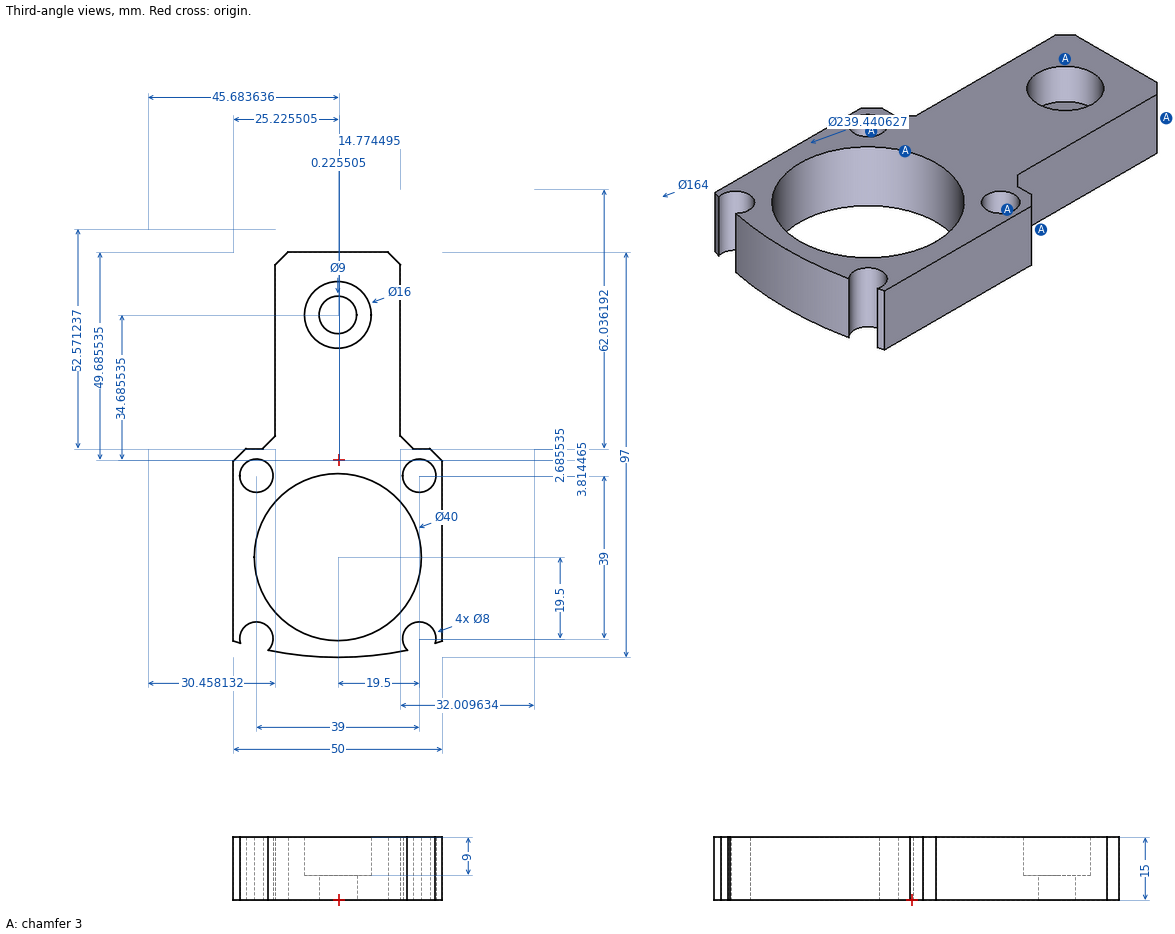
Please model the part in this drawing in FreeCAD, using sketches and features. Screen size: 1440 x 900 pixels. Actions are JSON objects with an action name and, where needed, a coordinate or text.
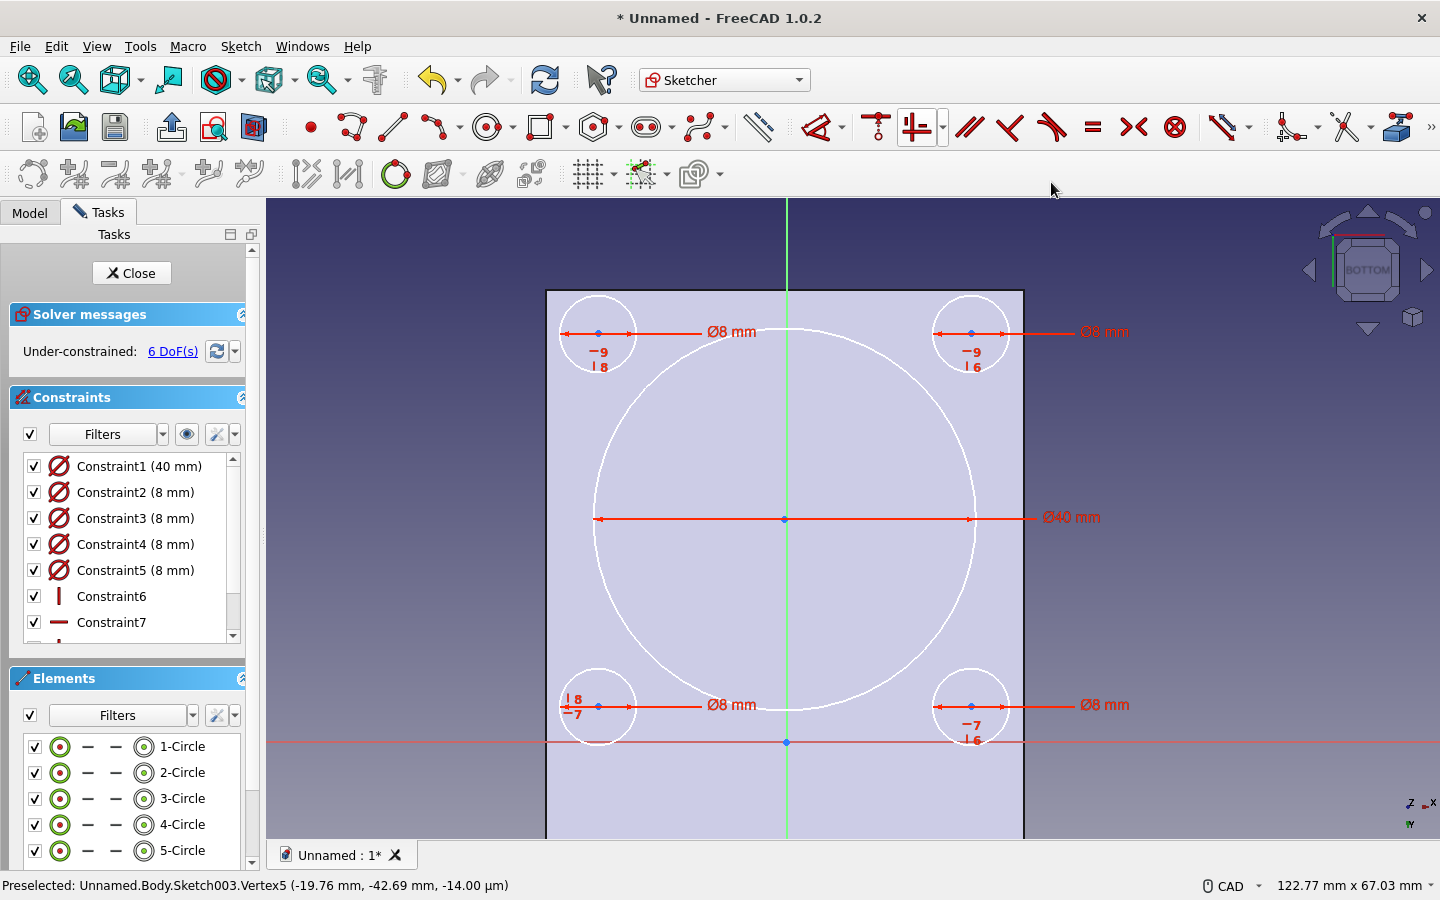
{"action": "left_click", "coordinate": [971, 334]}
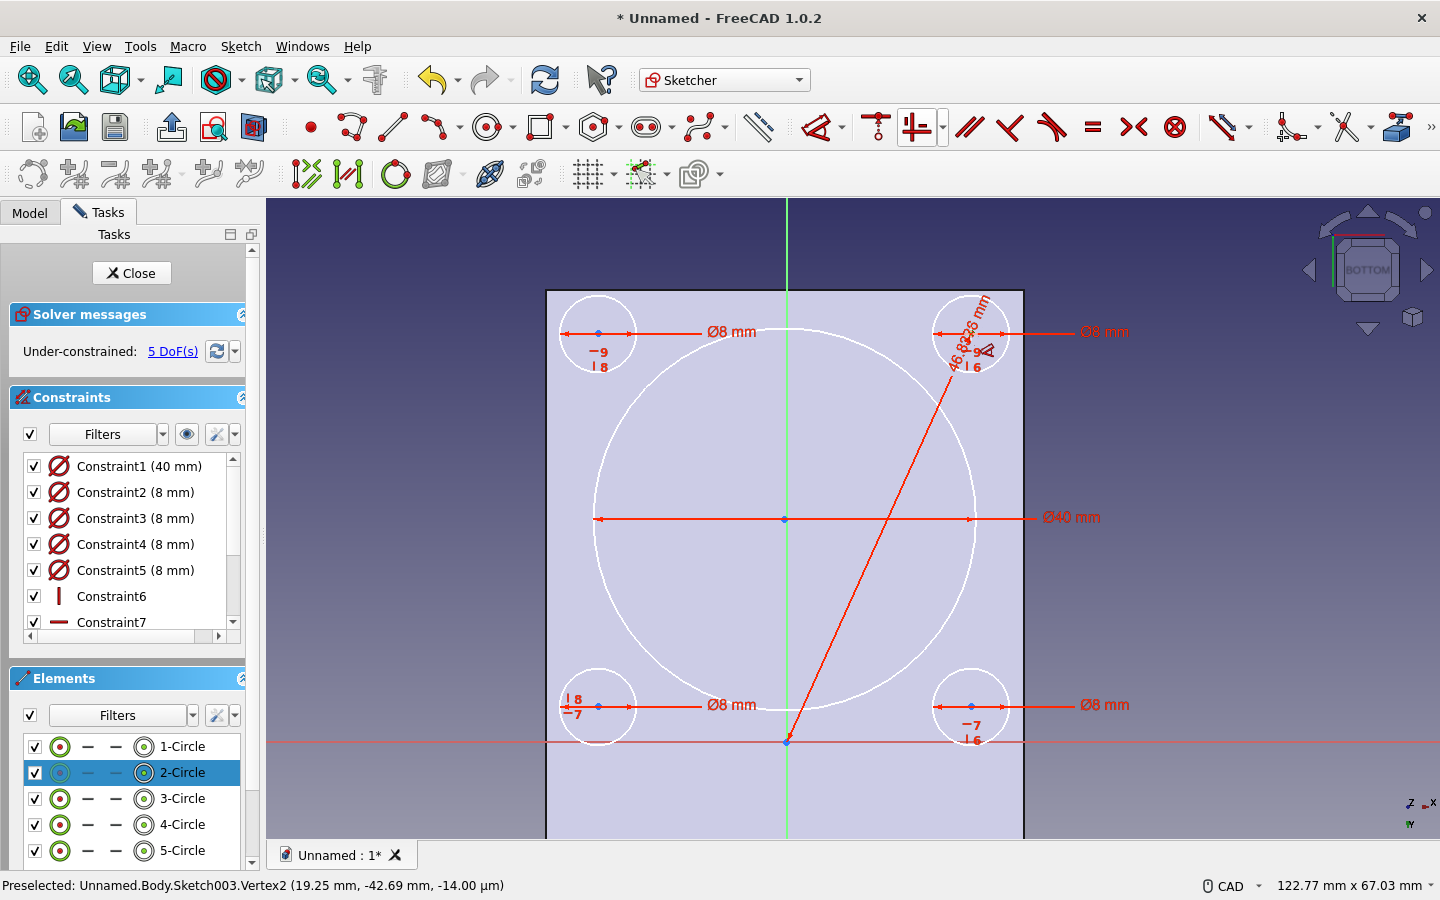
{"action": "left_click", "coordinate": [971, 707]}
{"action": "left_click", "coordinate": [1005, 521]}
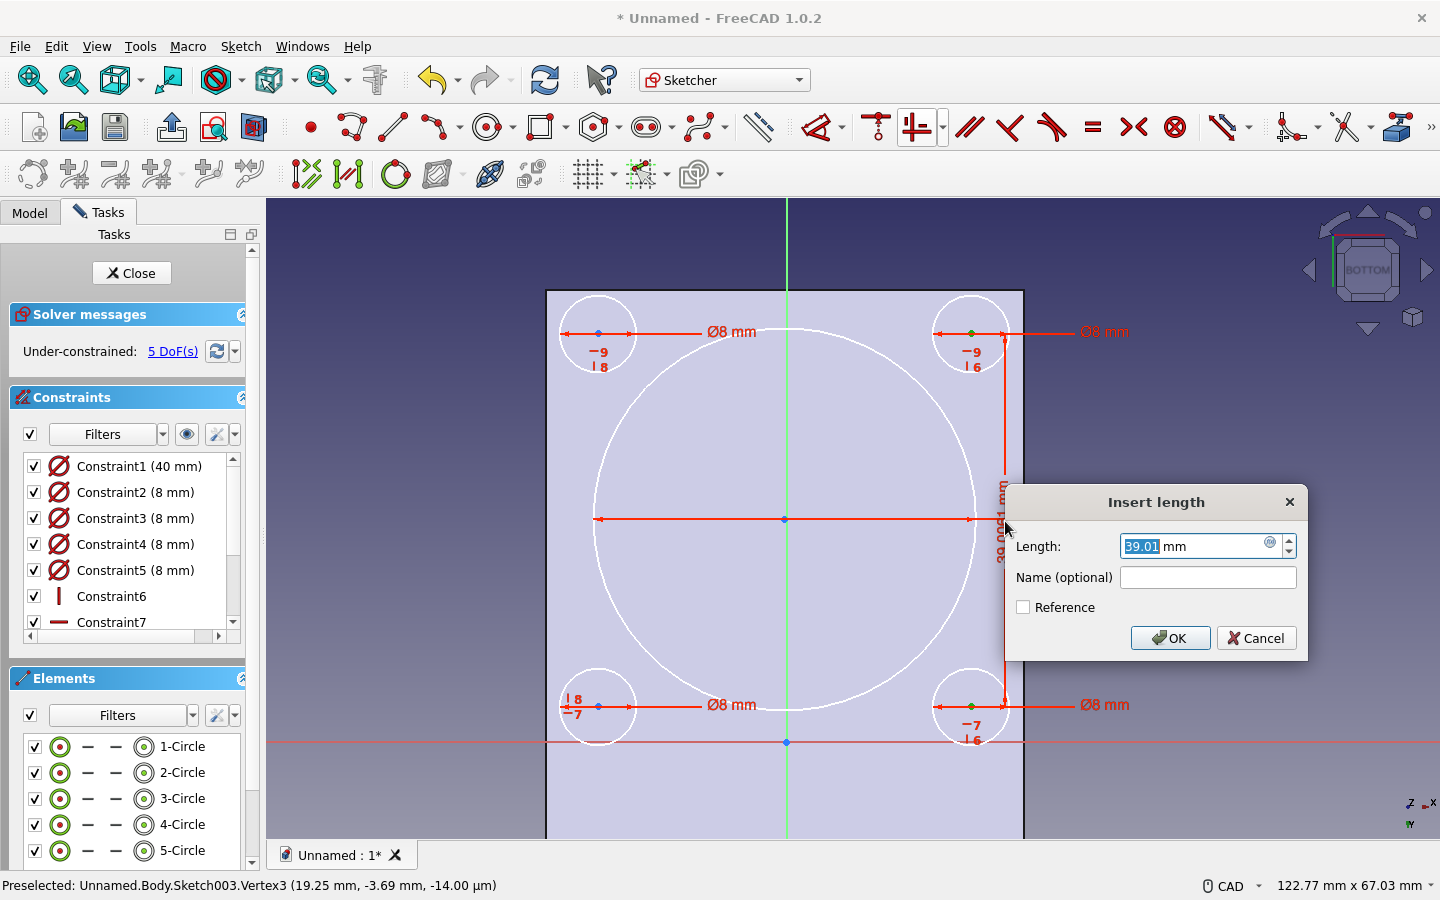
{"action": "type", "text": "39"}
{"action": "key", "text": "Return"}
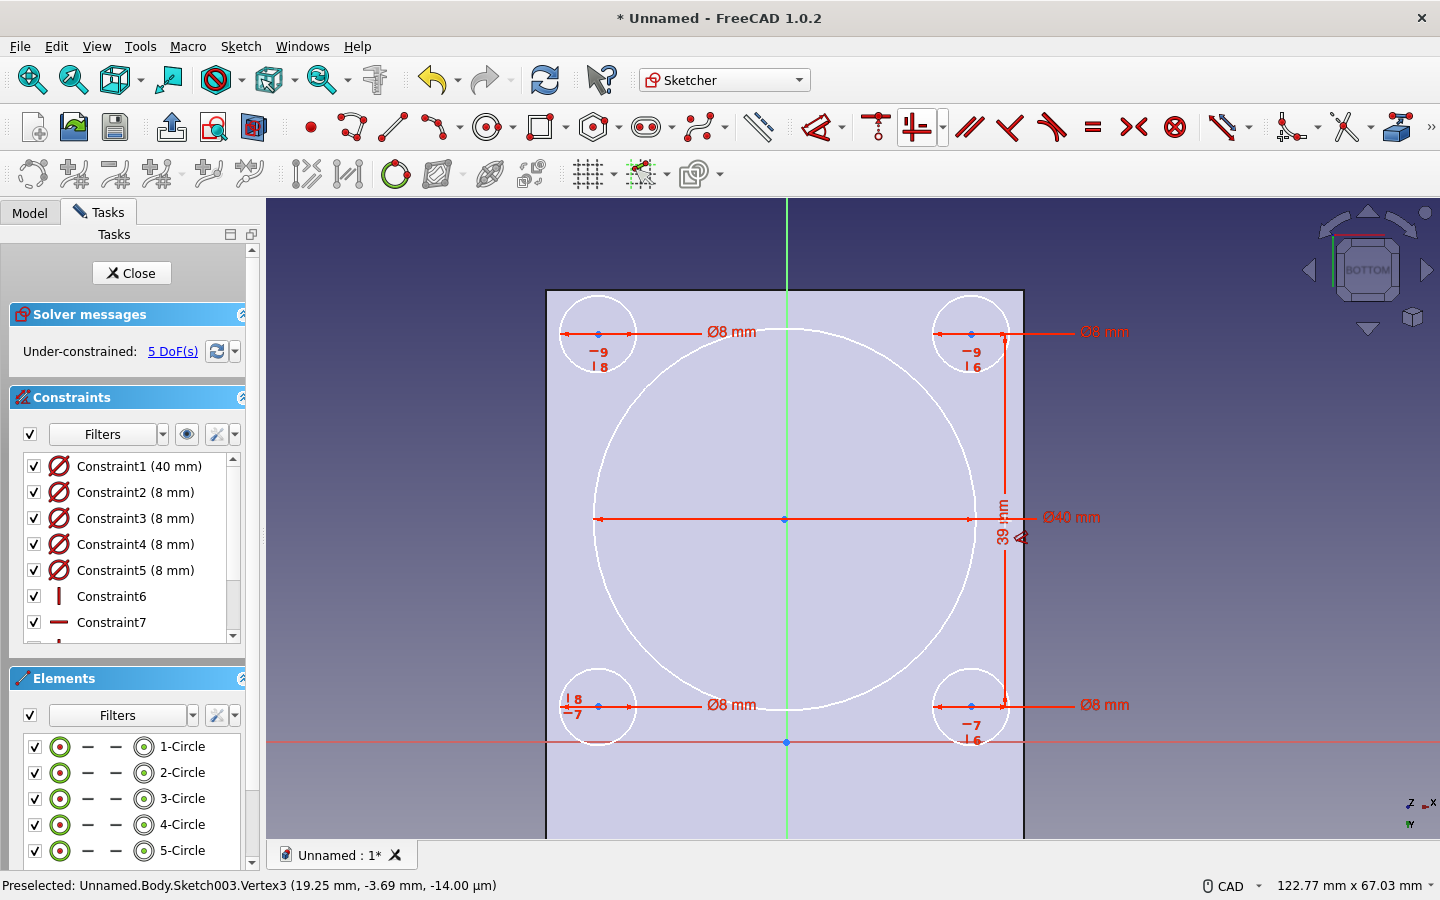
{"action": "left_click", "coordinate": [971, 707]}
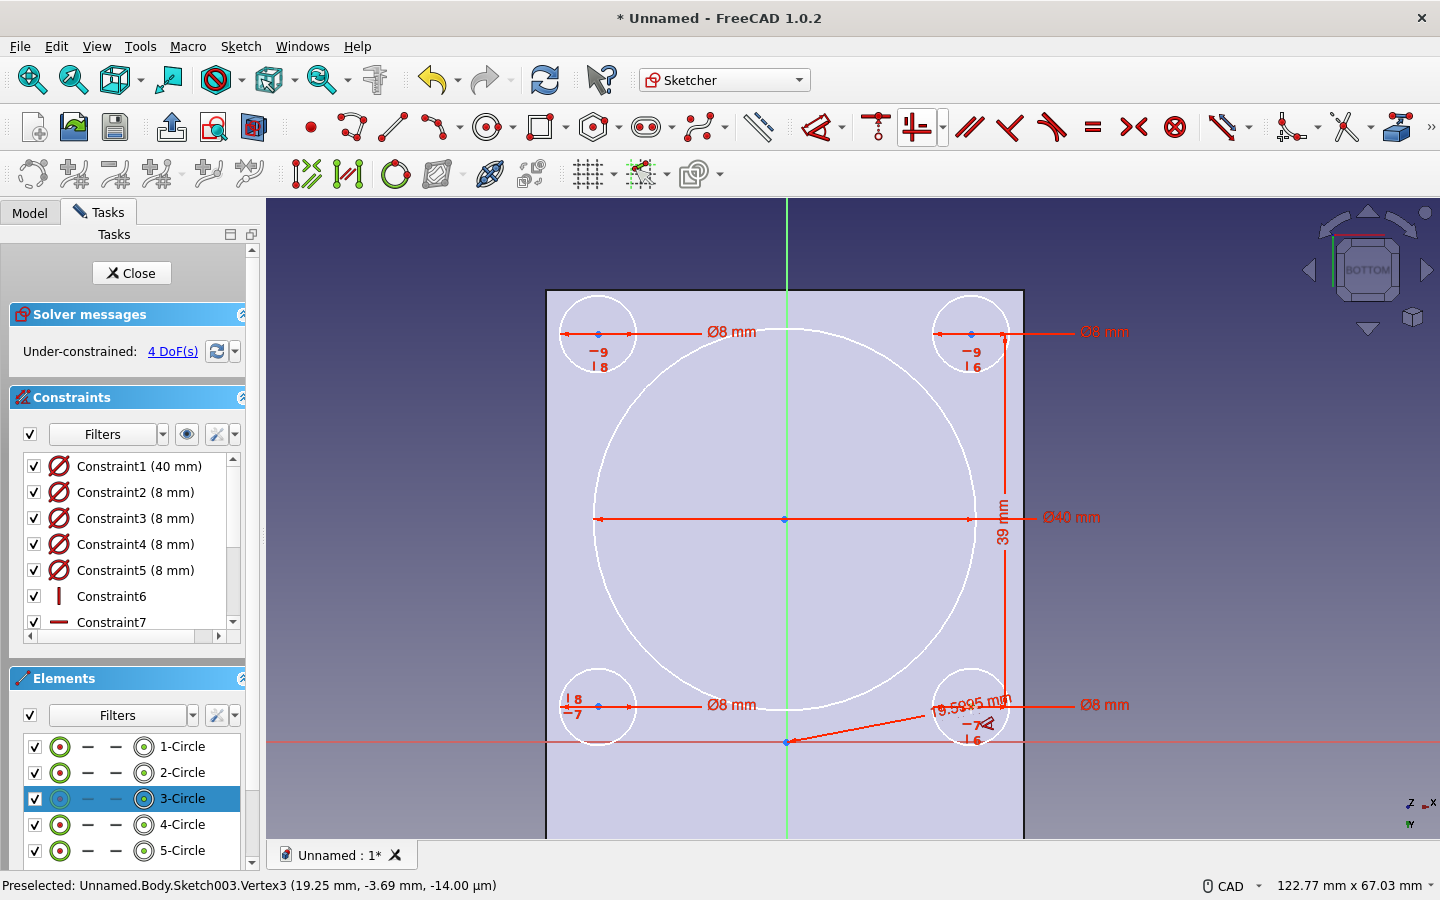
{"action": "left_click", "coordinate": [598, 707]}
{"action": "left_click", "coordinate": [699, 673]}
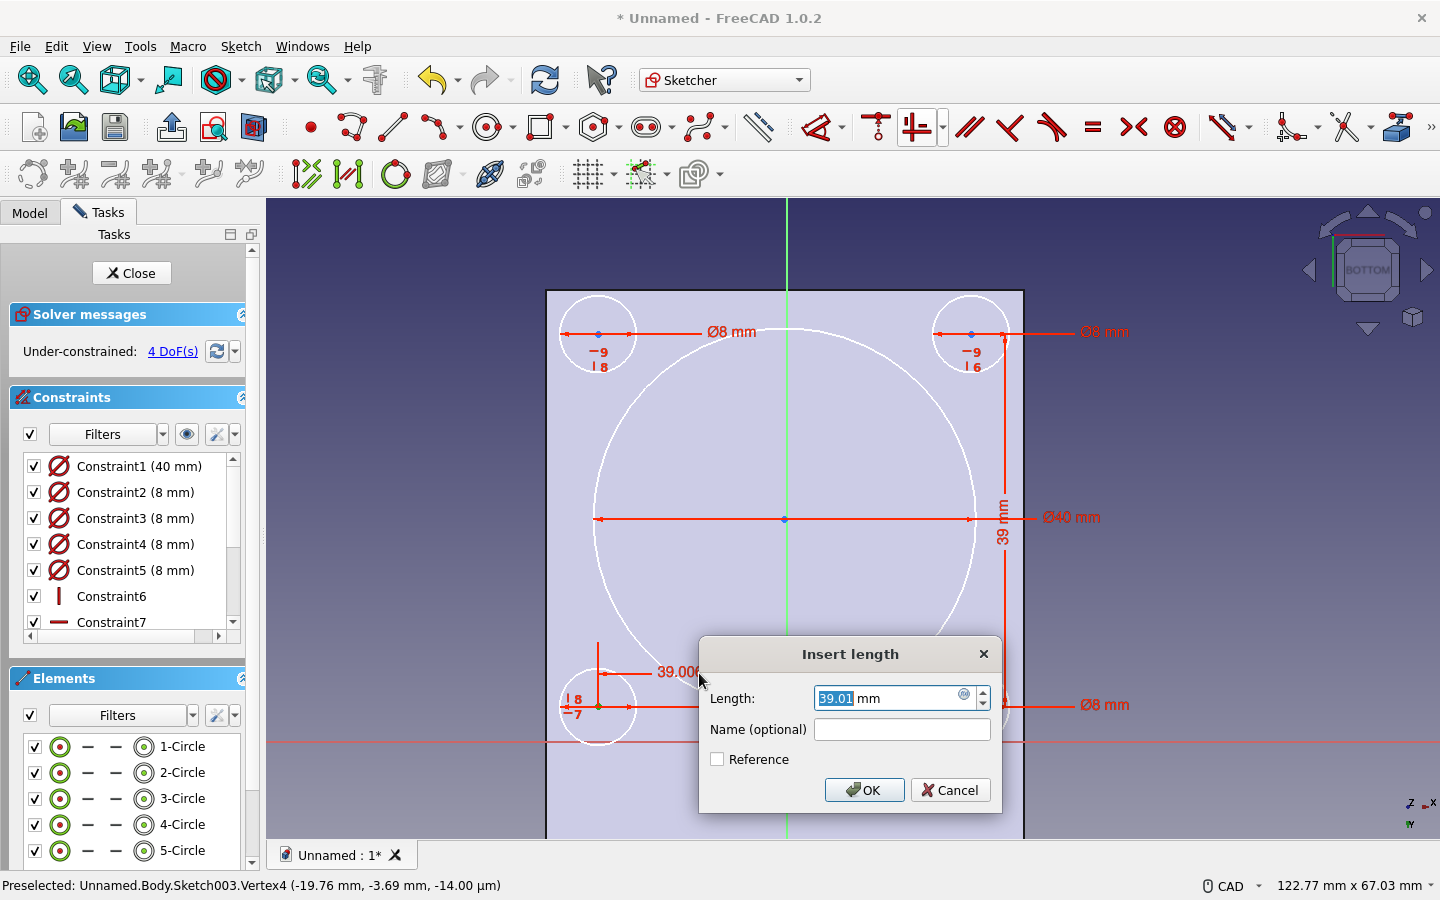
{"action": "type", "text": "39"}
{"action": "key", "text": "Return"}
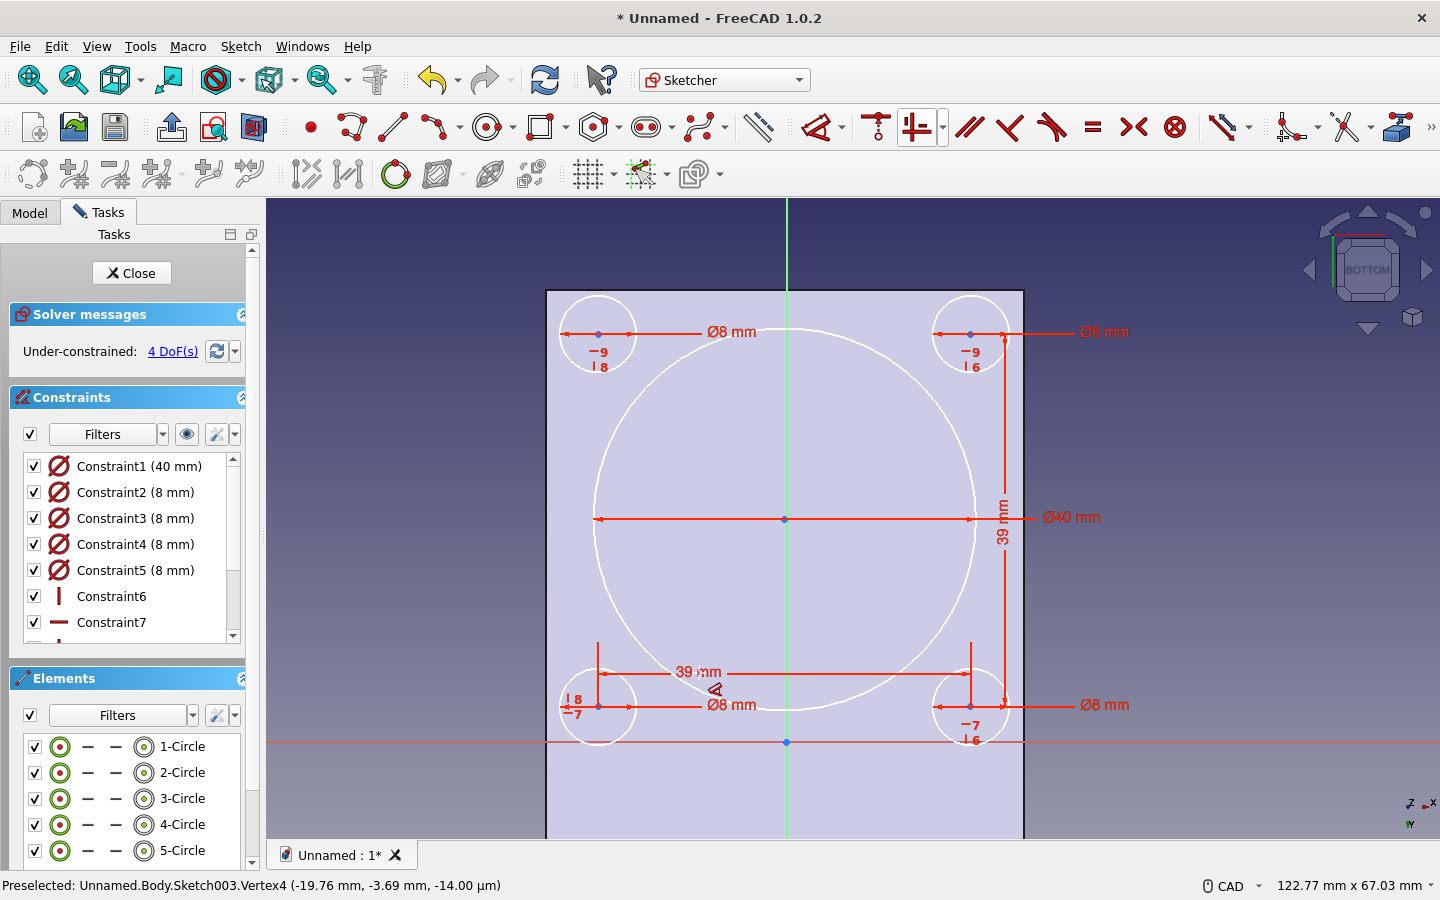
{"action": "left_click", "coordinate": [785, 519]}